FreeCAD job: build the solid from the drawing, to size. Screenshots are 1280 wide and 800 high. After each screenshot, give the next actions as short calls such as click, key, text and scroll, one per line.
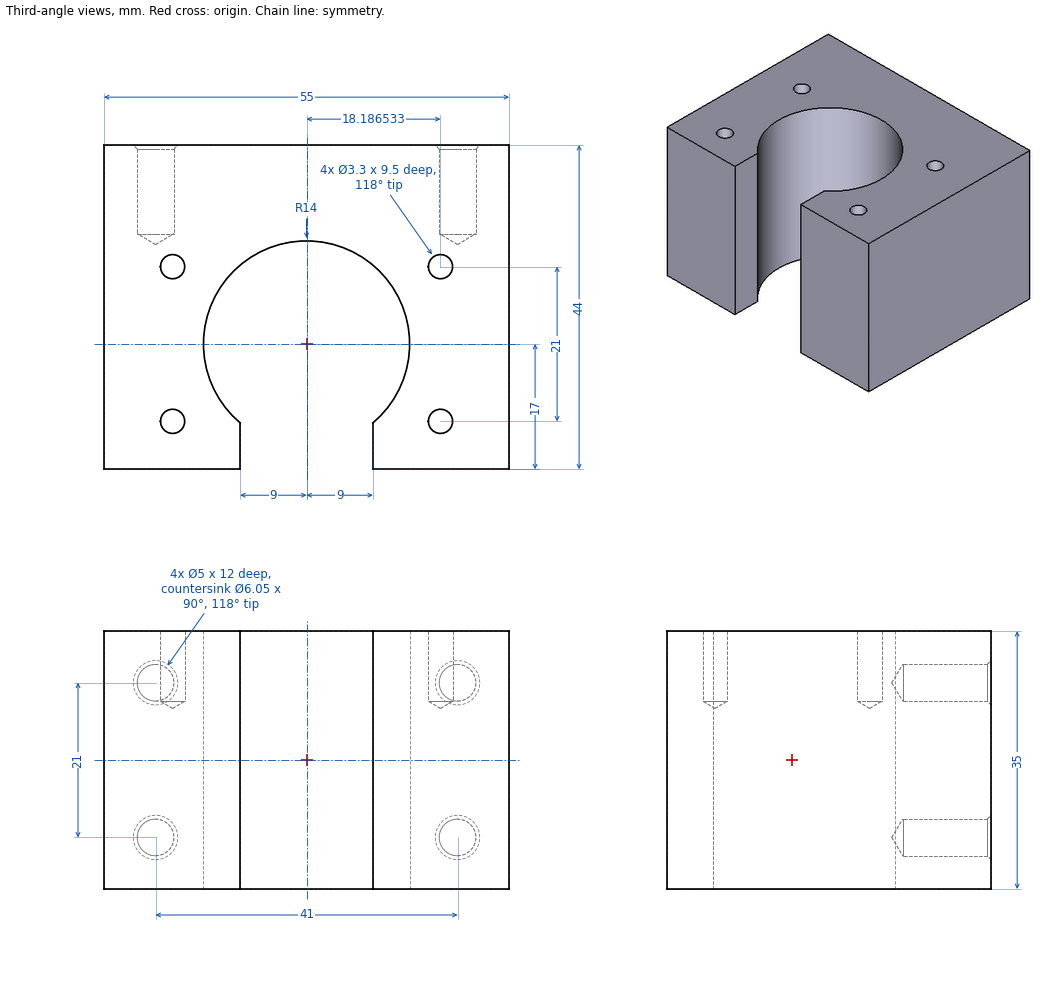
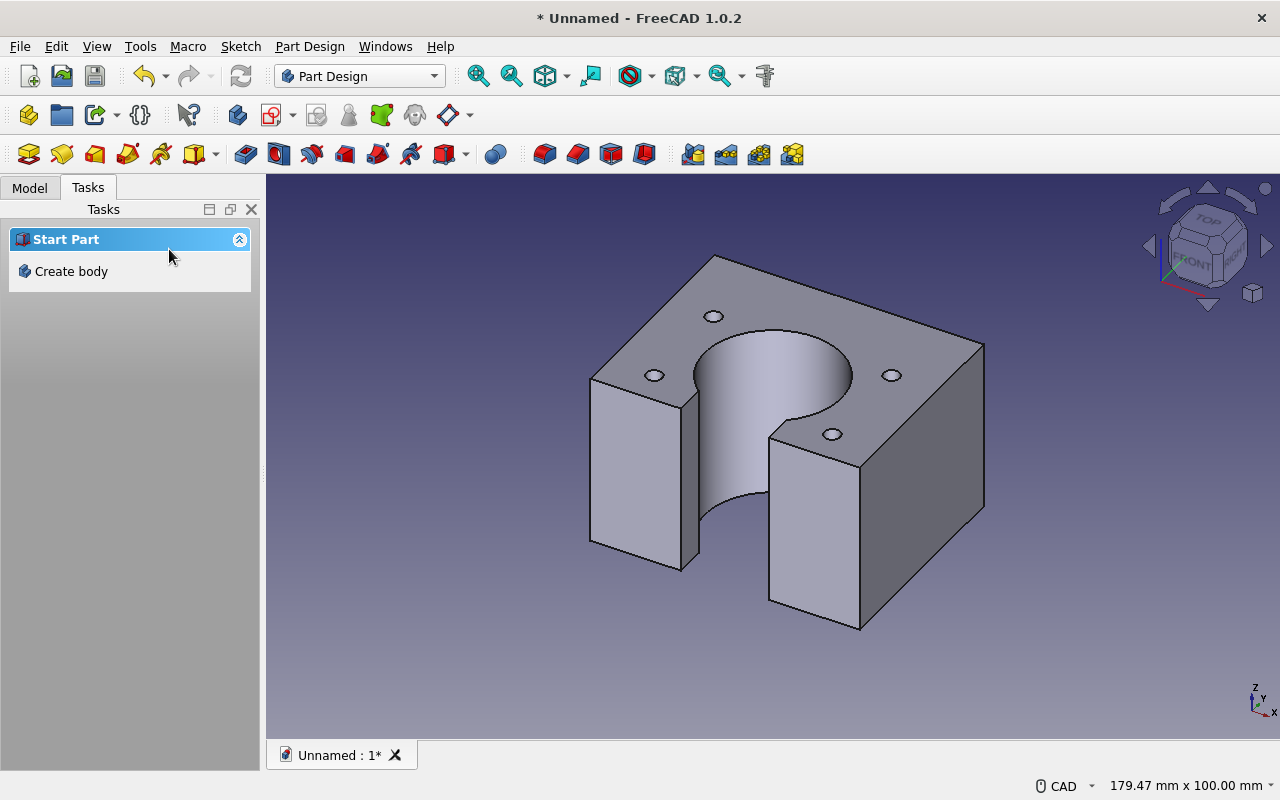
key(4)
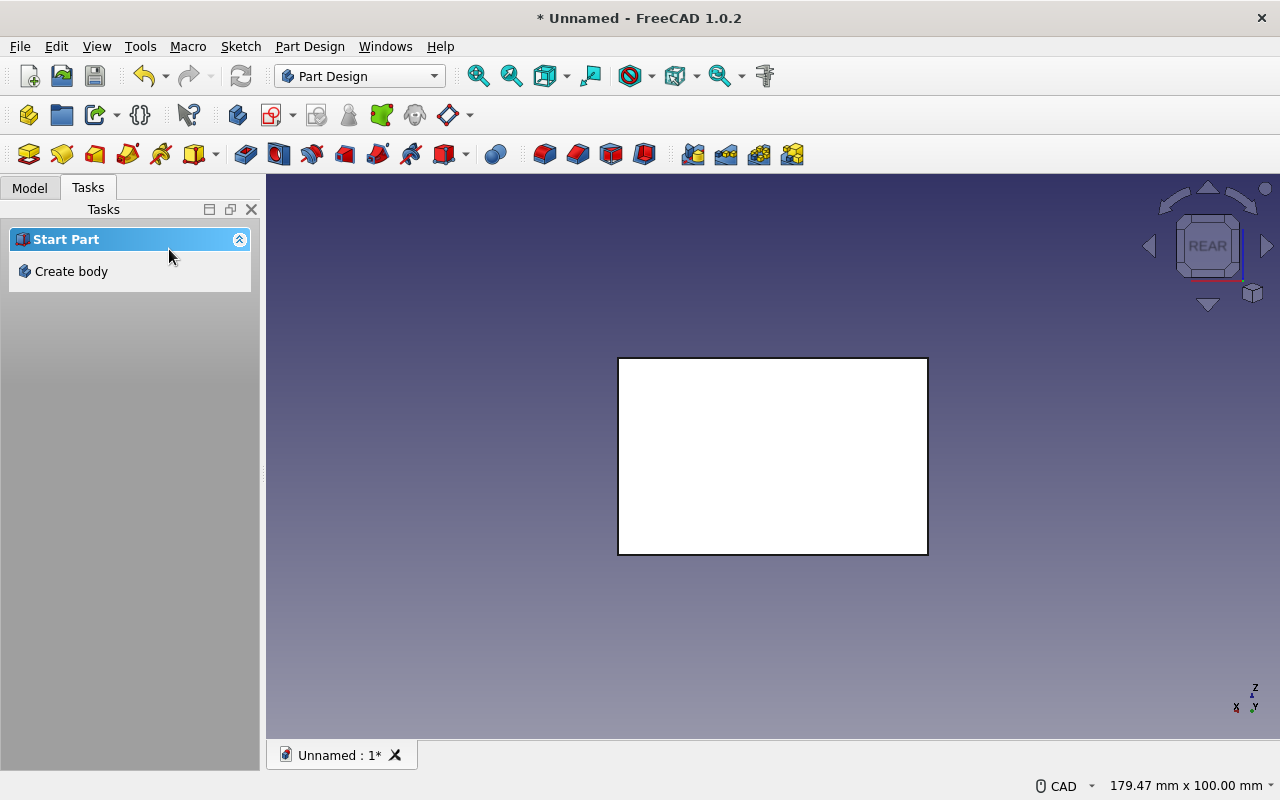
click(479, 76)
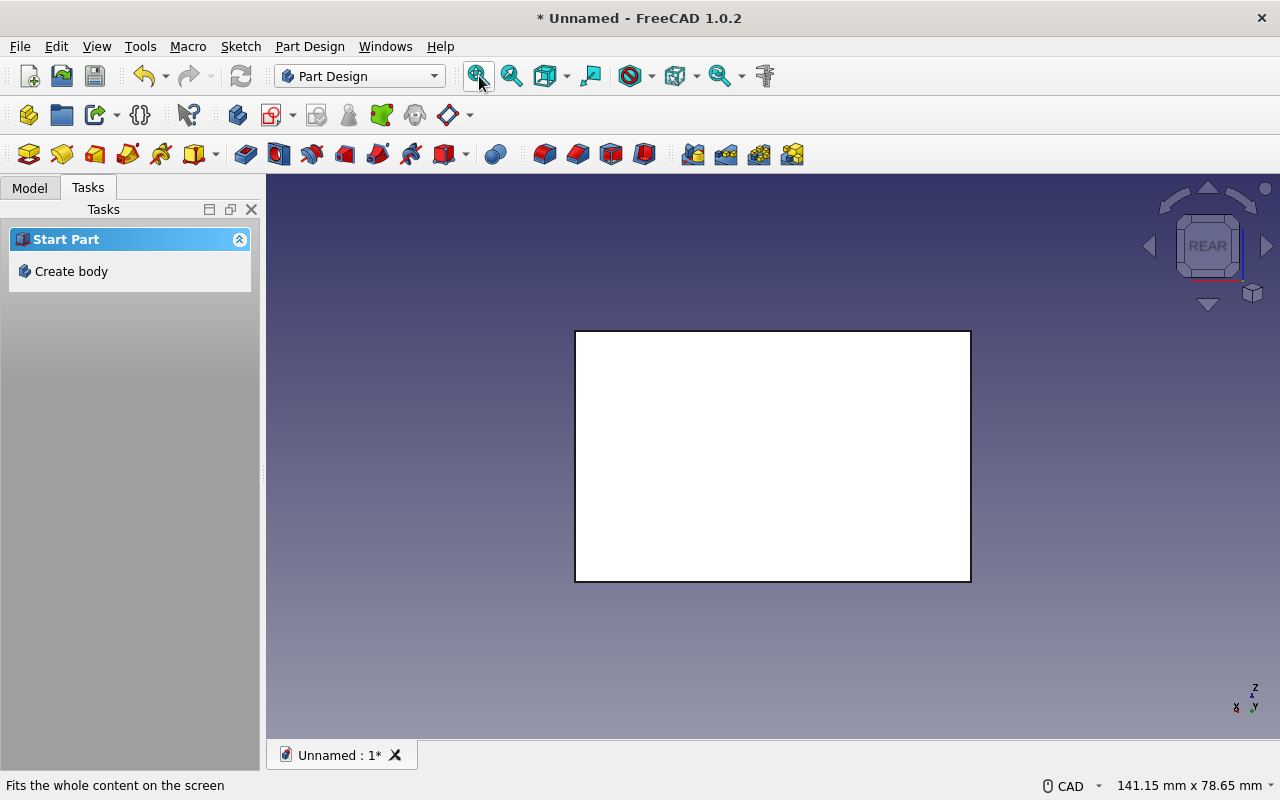
click(717, 456)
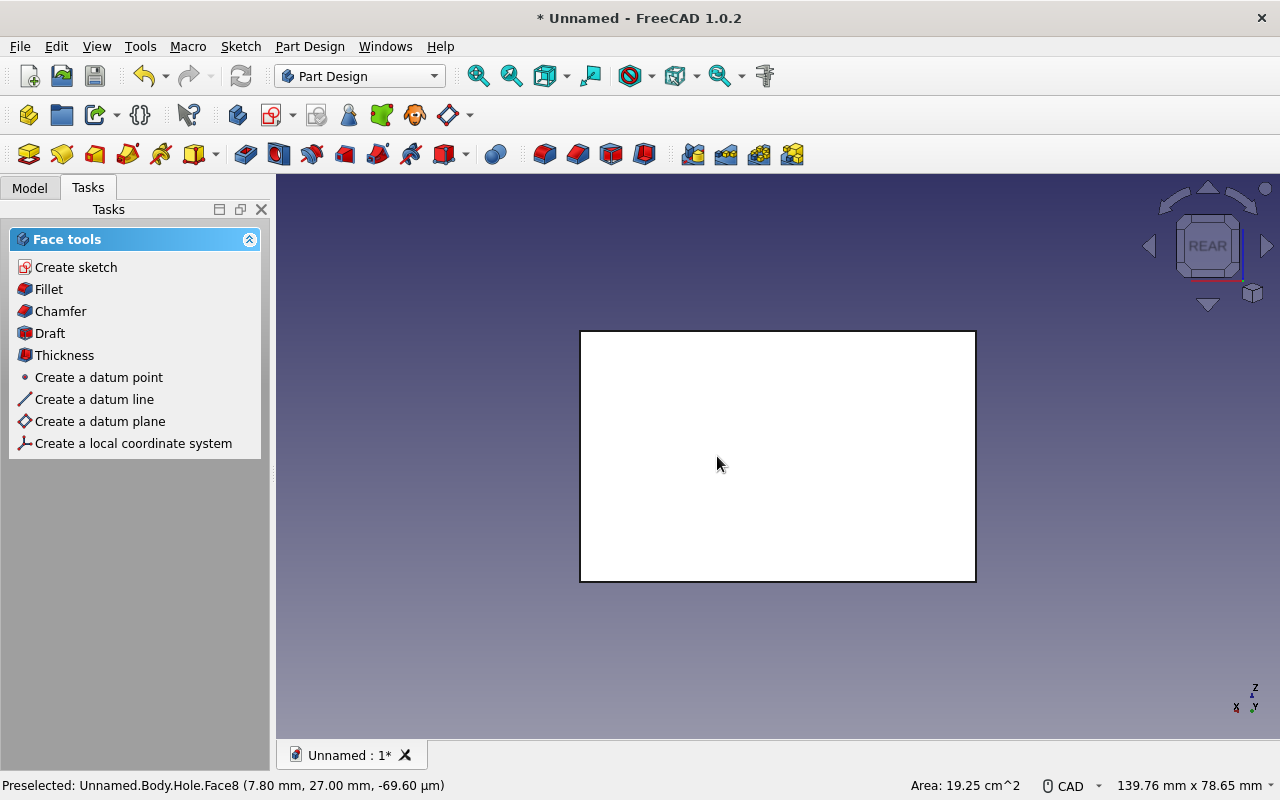
click(270, 116)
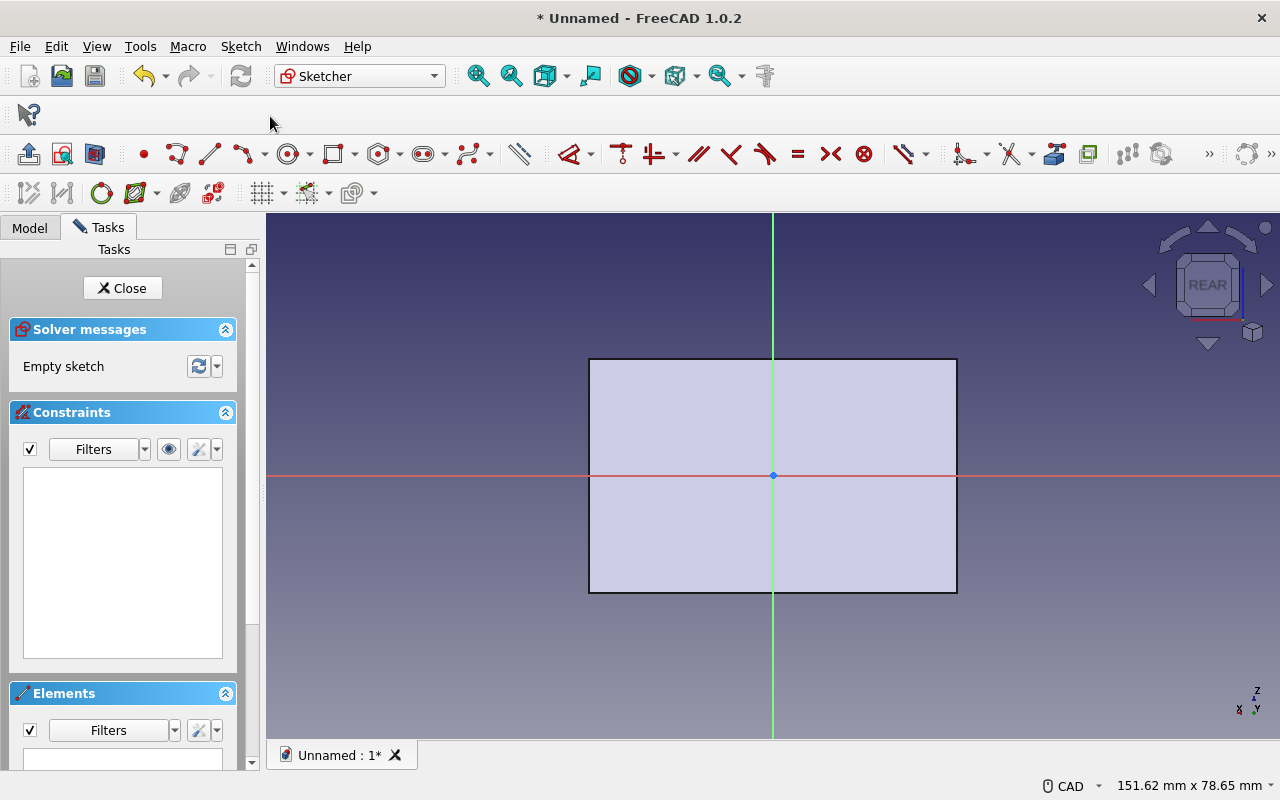
scroll(856, 476, up, 3)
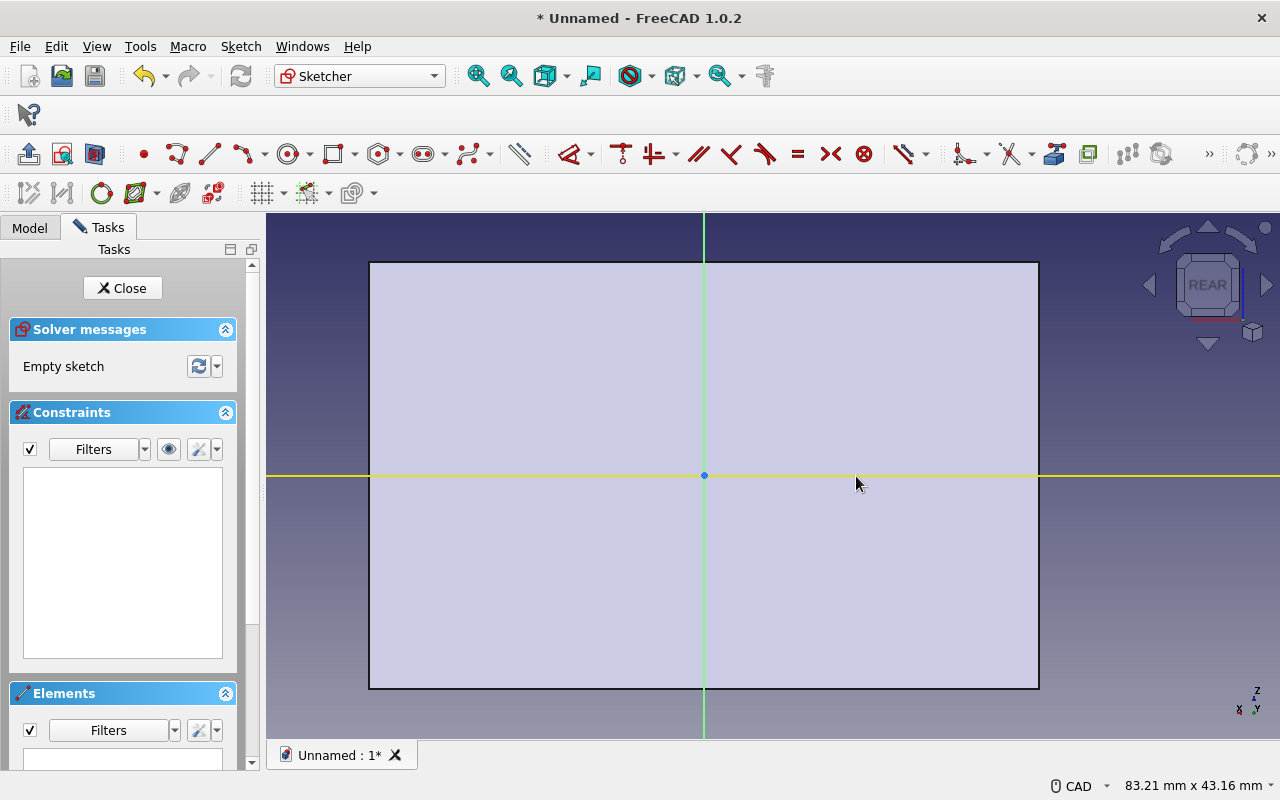
click(288, 154)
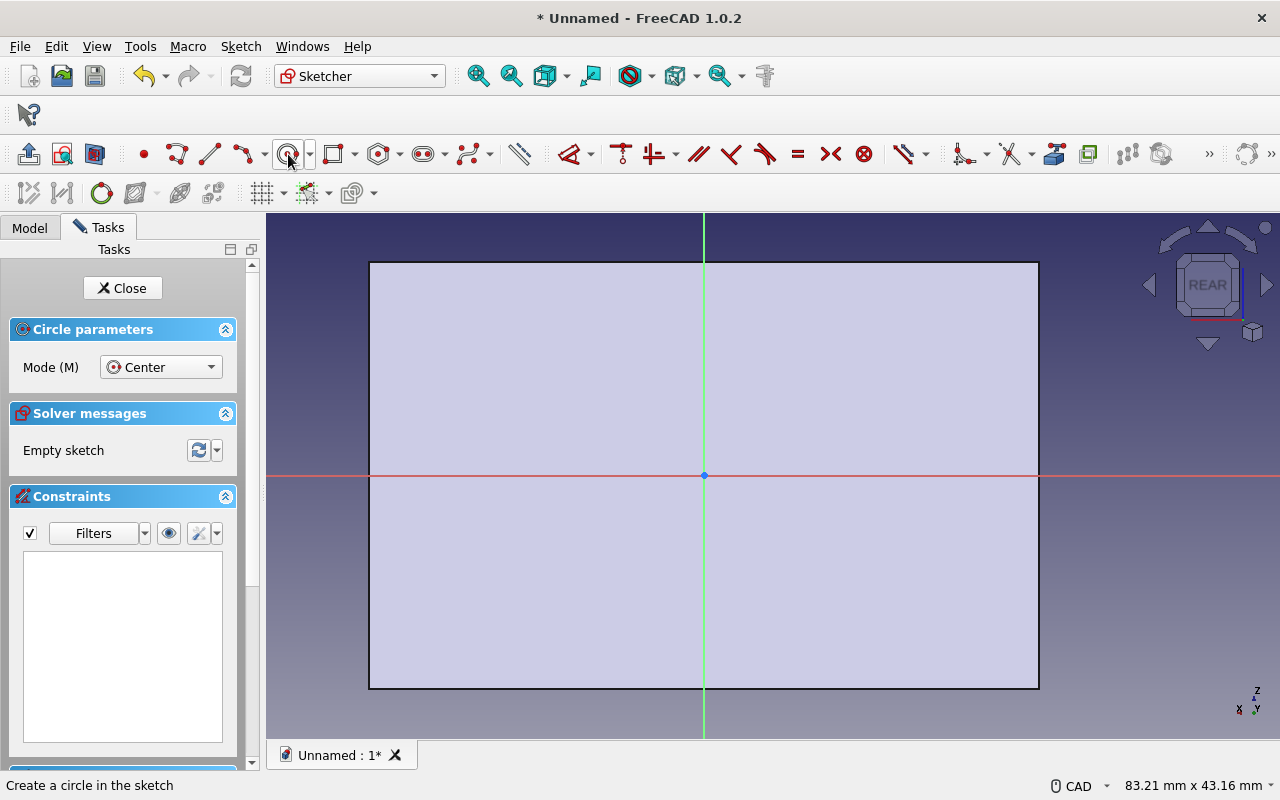
click(954, 348)
move(976, 326)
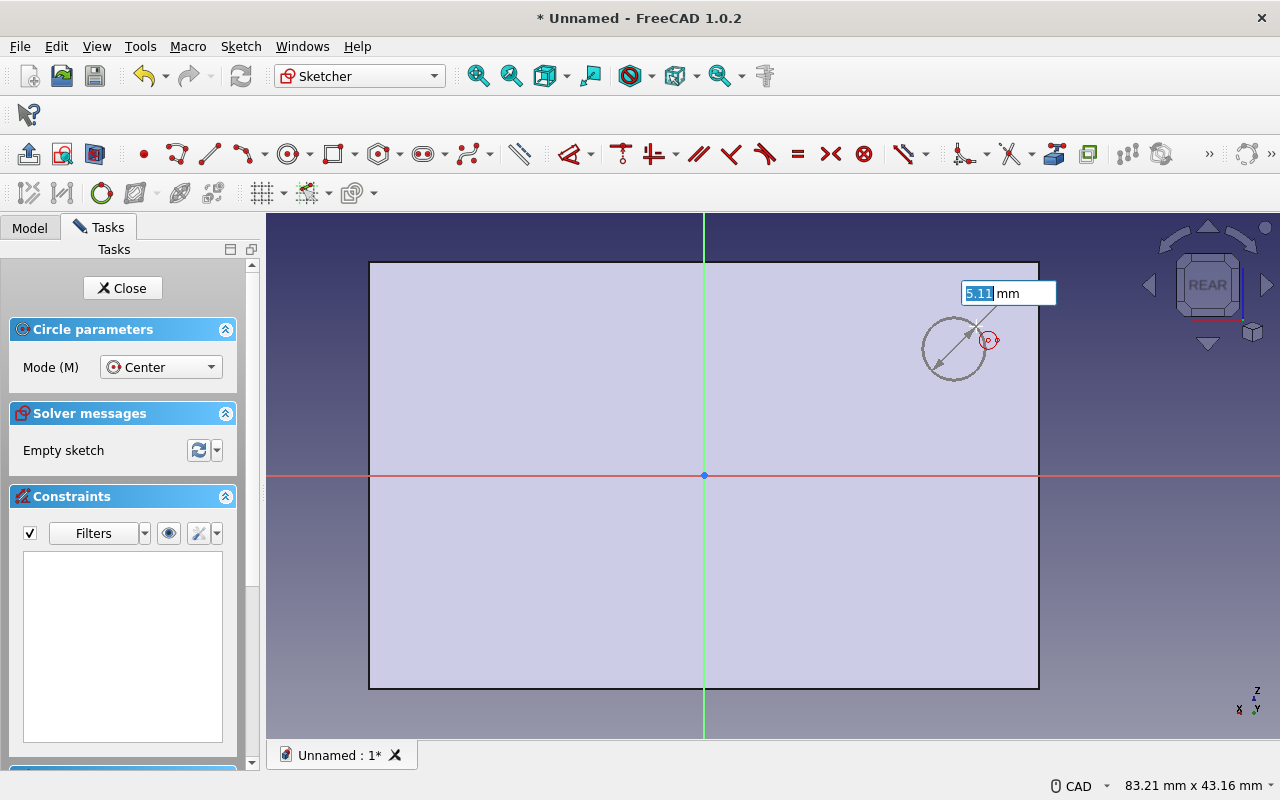
text(5)
key(Return)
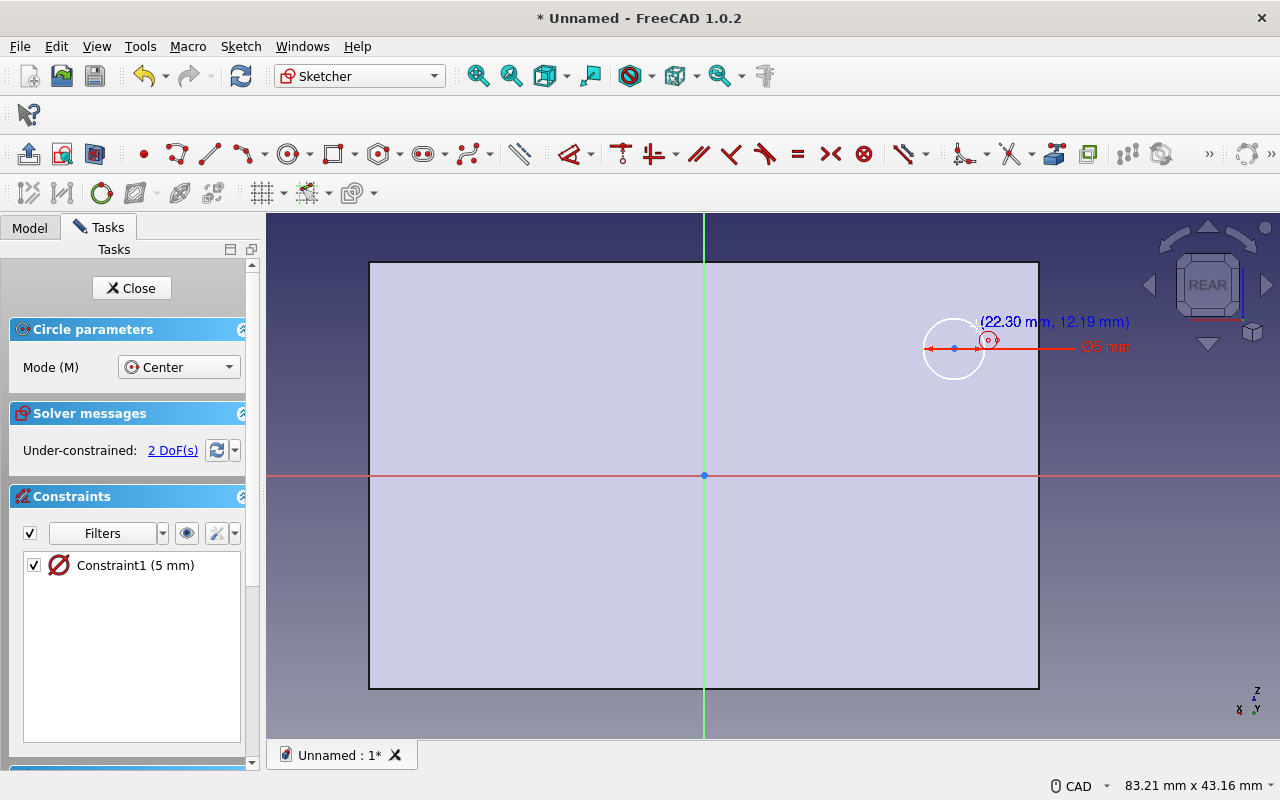
click(954, 604)
move(976, 582)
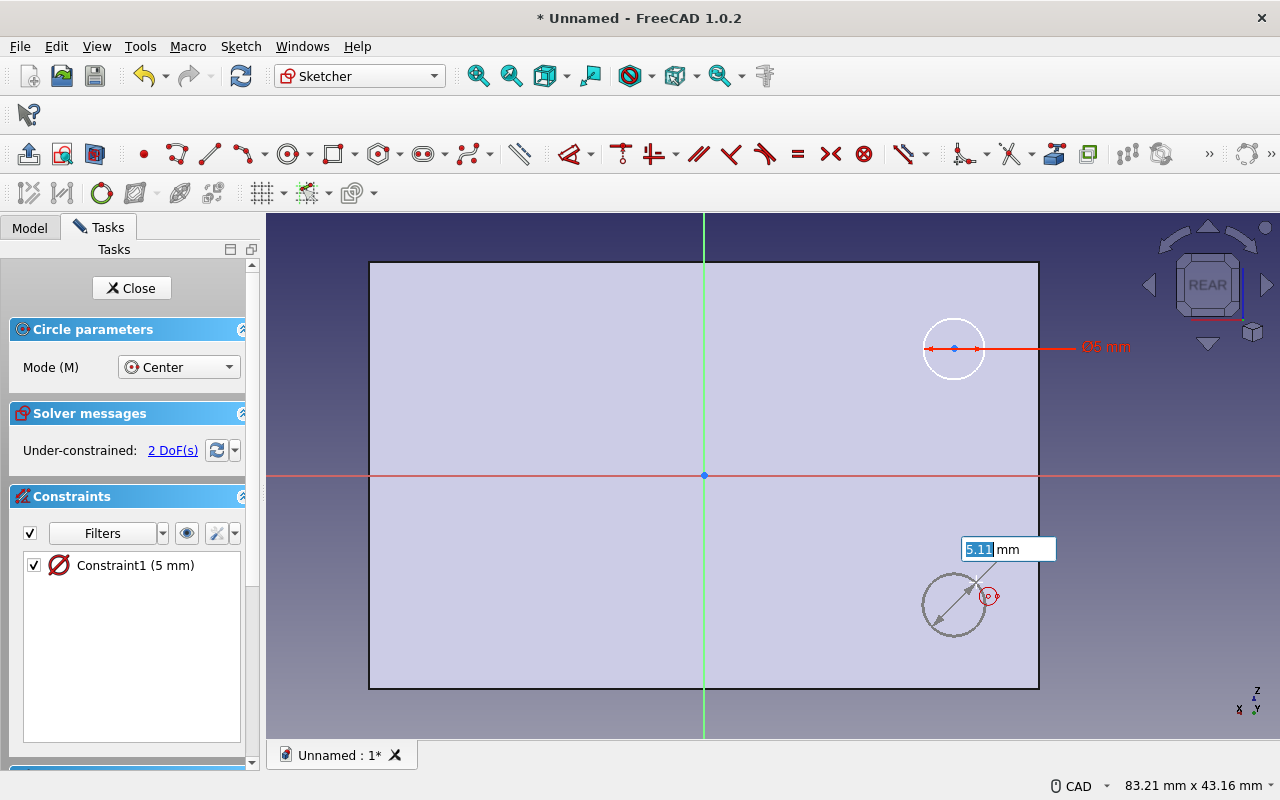
text(5)
key(Return)